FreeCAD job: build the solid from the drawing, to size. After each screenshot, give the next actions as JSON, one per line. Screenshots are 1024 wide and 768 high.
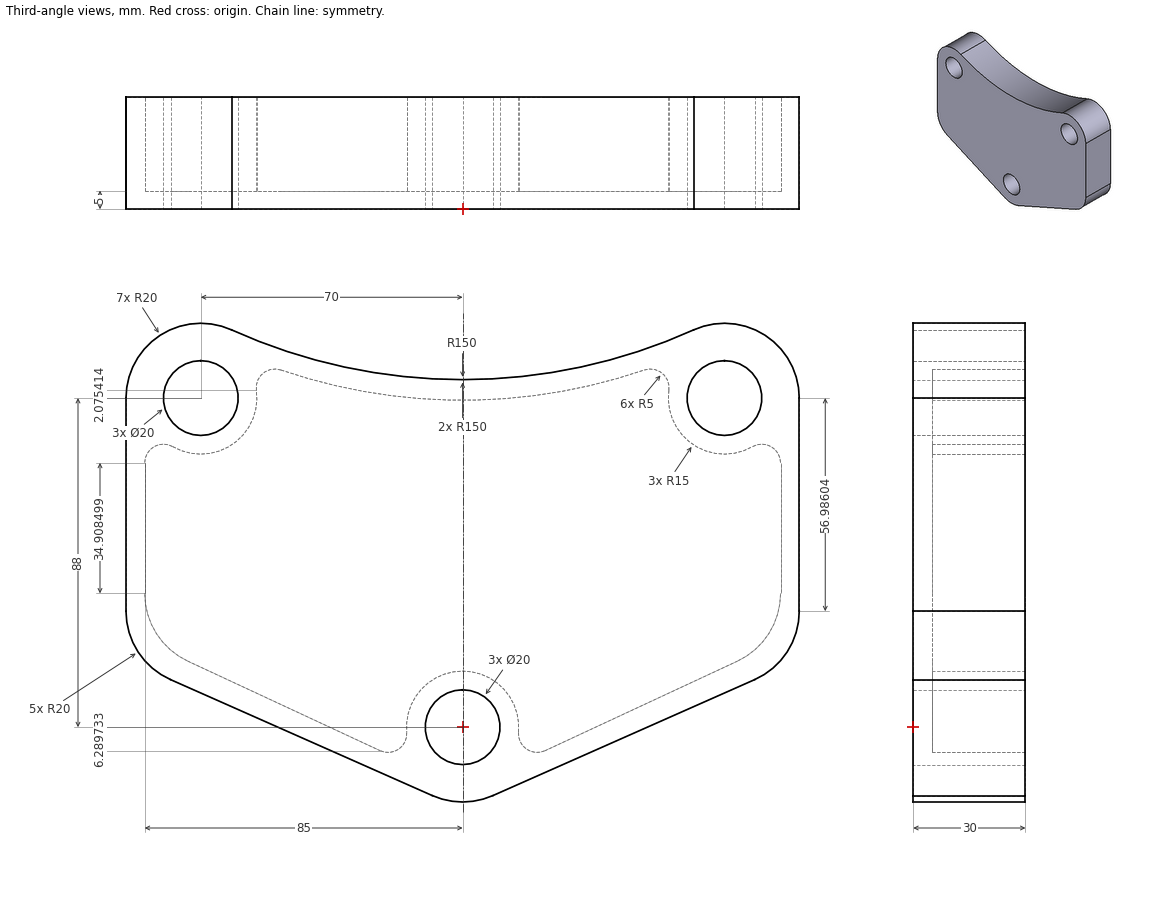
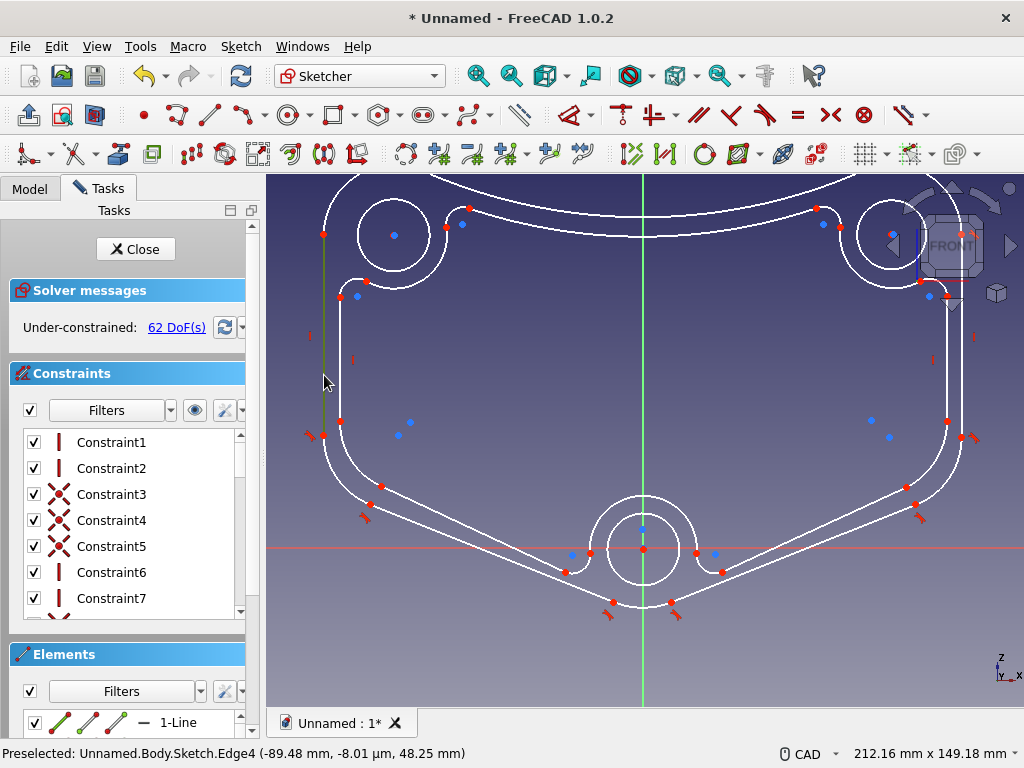
{"action": "left_click", "coordinate": [329, 208]}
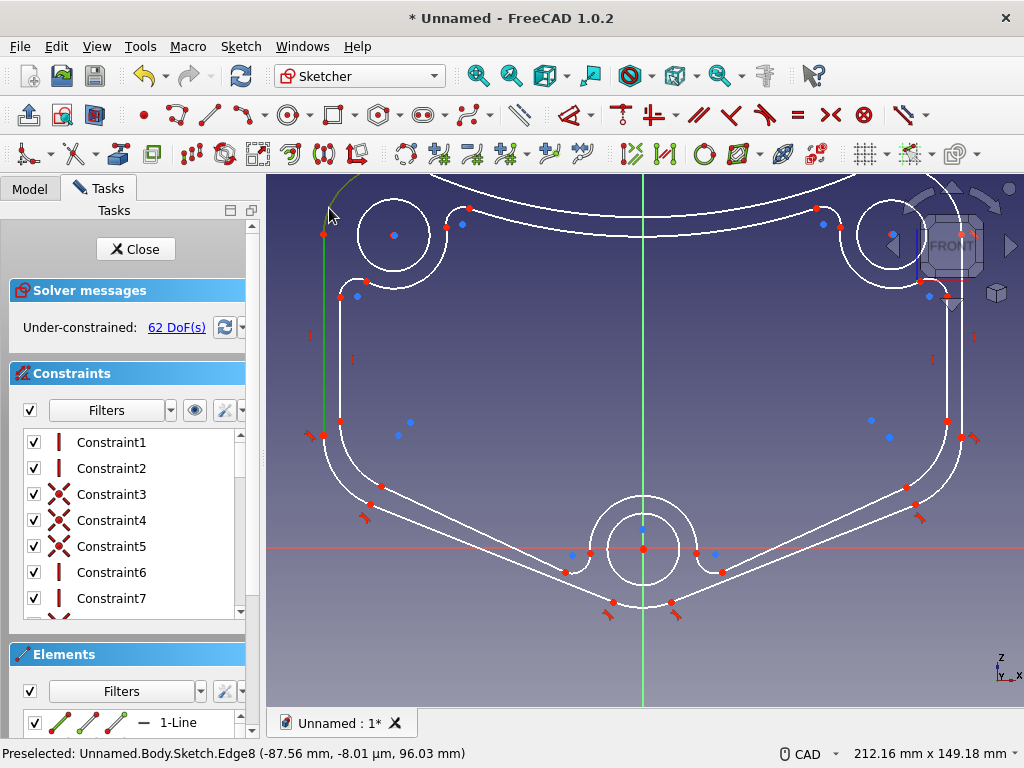
{"action": "left_click", "coordinate": [765, 116]}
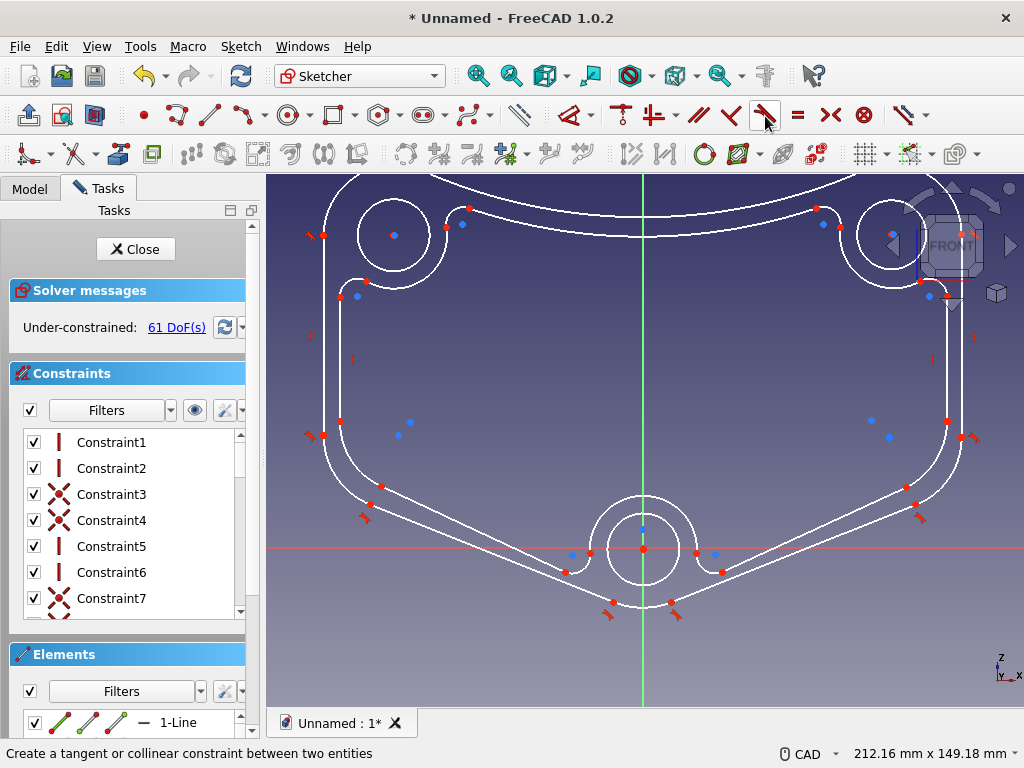
{"action": "left_click", "coordinate": [329, 209]}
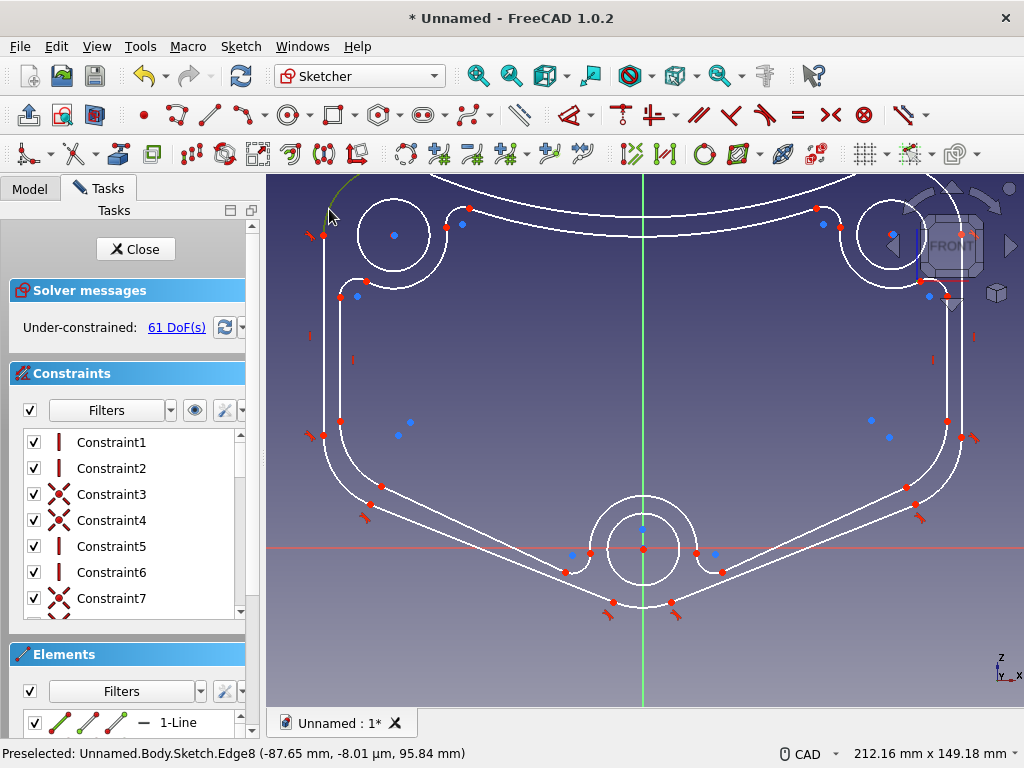
{"action": "left_click", "coordinate": [552, 210]}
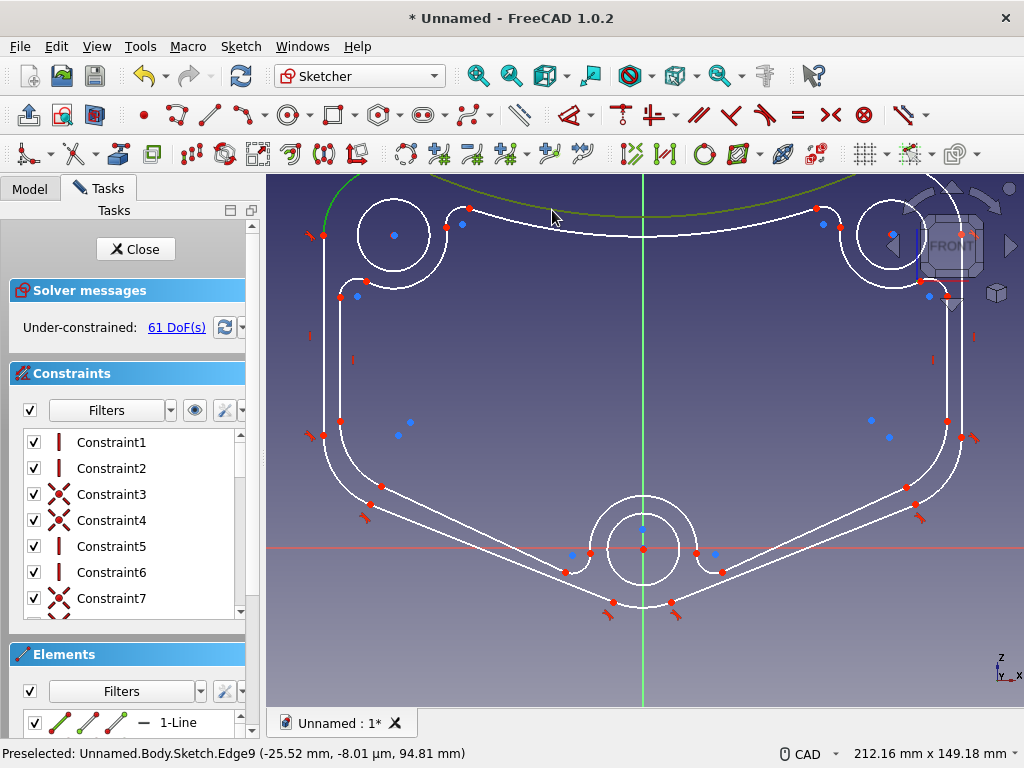
{"action": "left_click", "coordinate": [765, 116]}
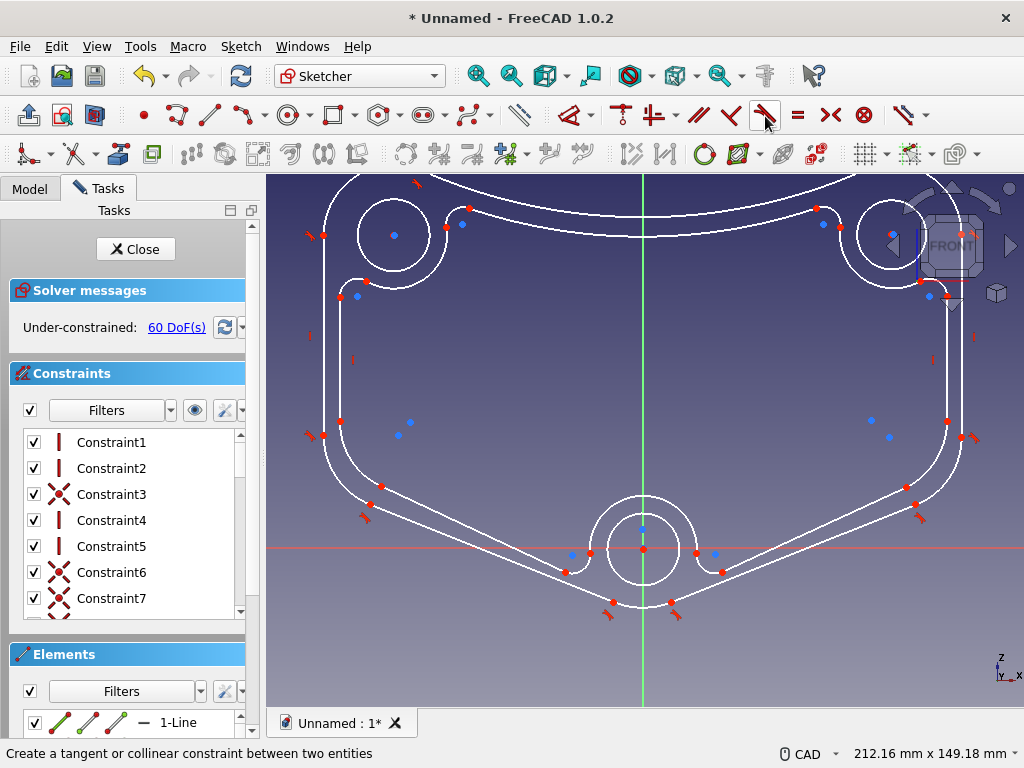
{"action": "left_click", "coordinate": [553, 210]}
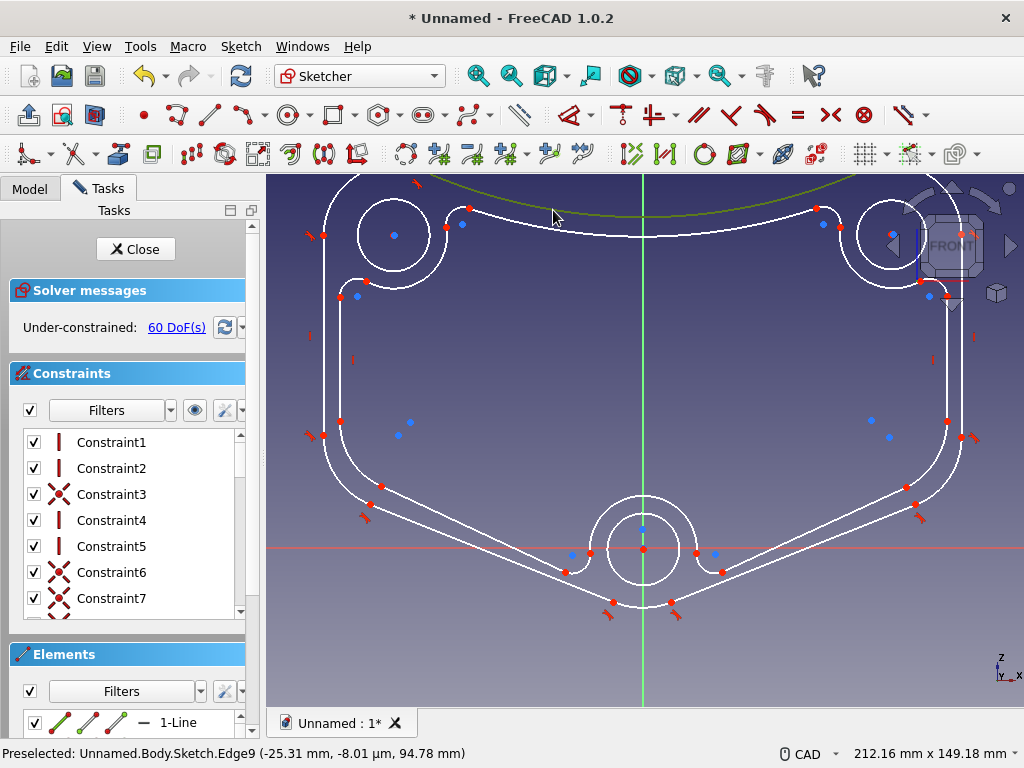
{"action": "scroll", "coordinate": [440, 534], "scroll_direction": "down", "scroll_amount": 2}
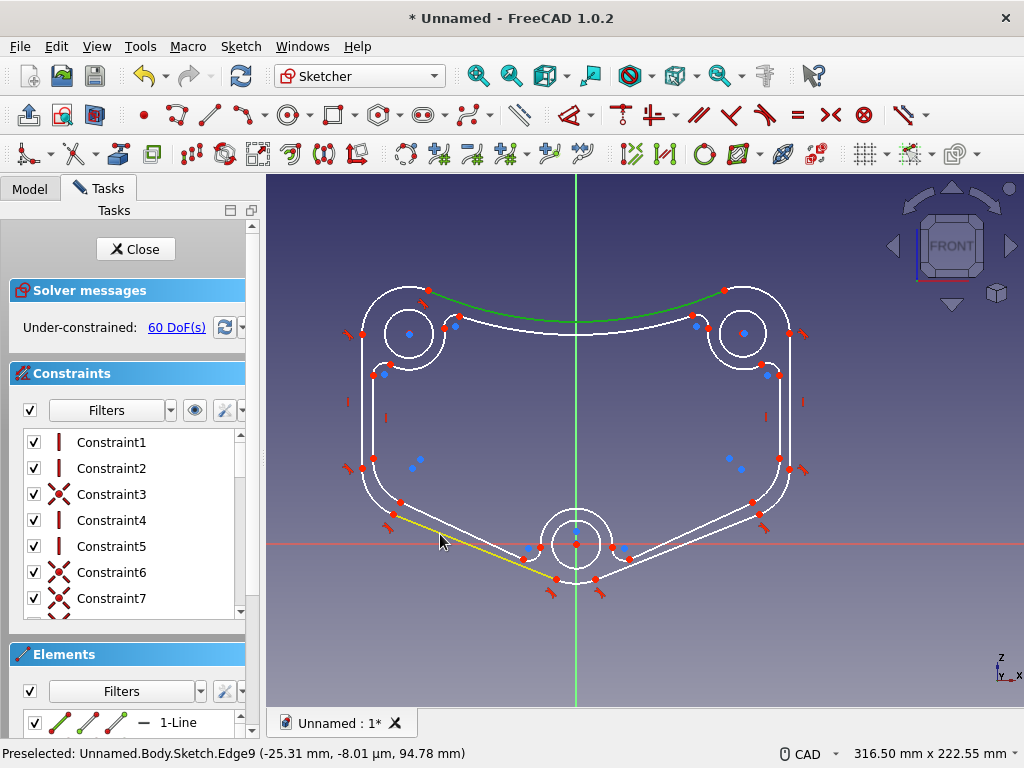
{"action": "left_click", "coordinate": [782, 307]}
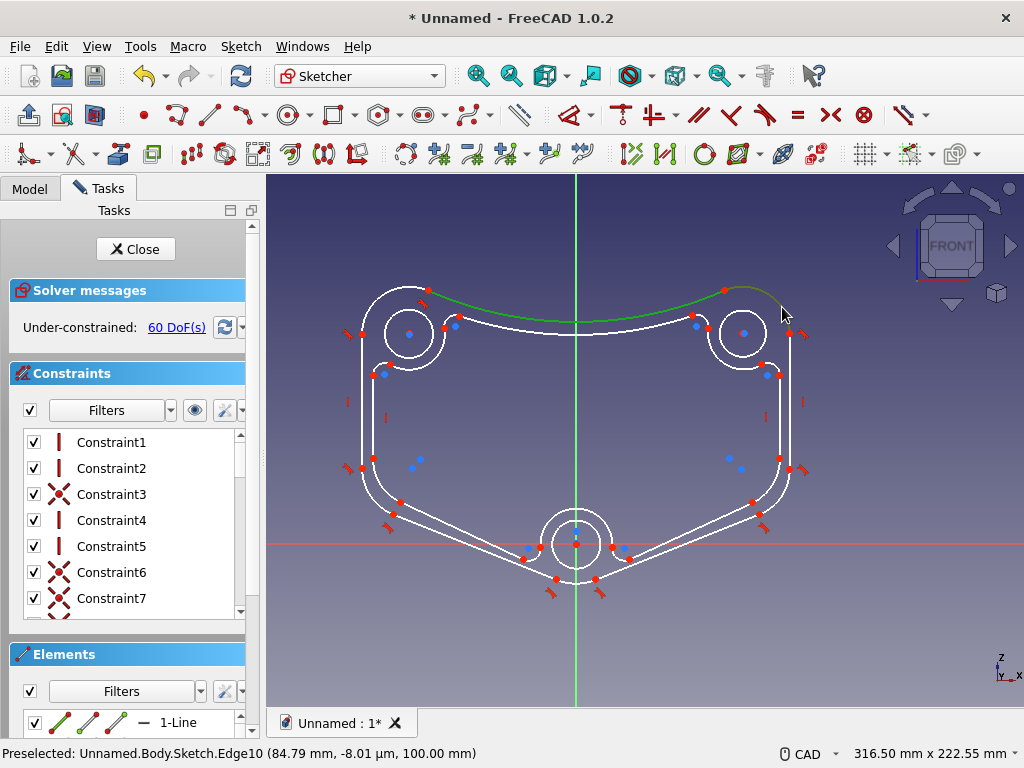
{"action": "left_click", "coordinate": [765, 116]}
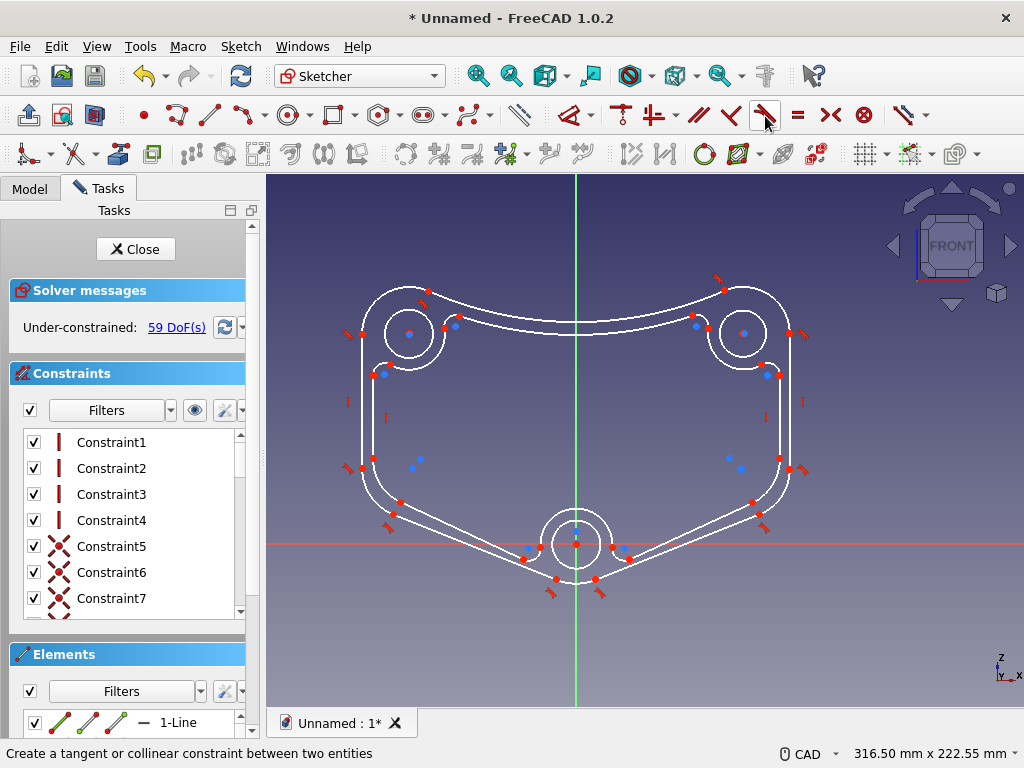
{"action": "scroll", "coordinate": [373, 400], "scroll_direction": "up", "scroll_amount": 2}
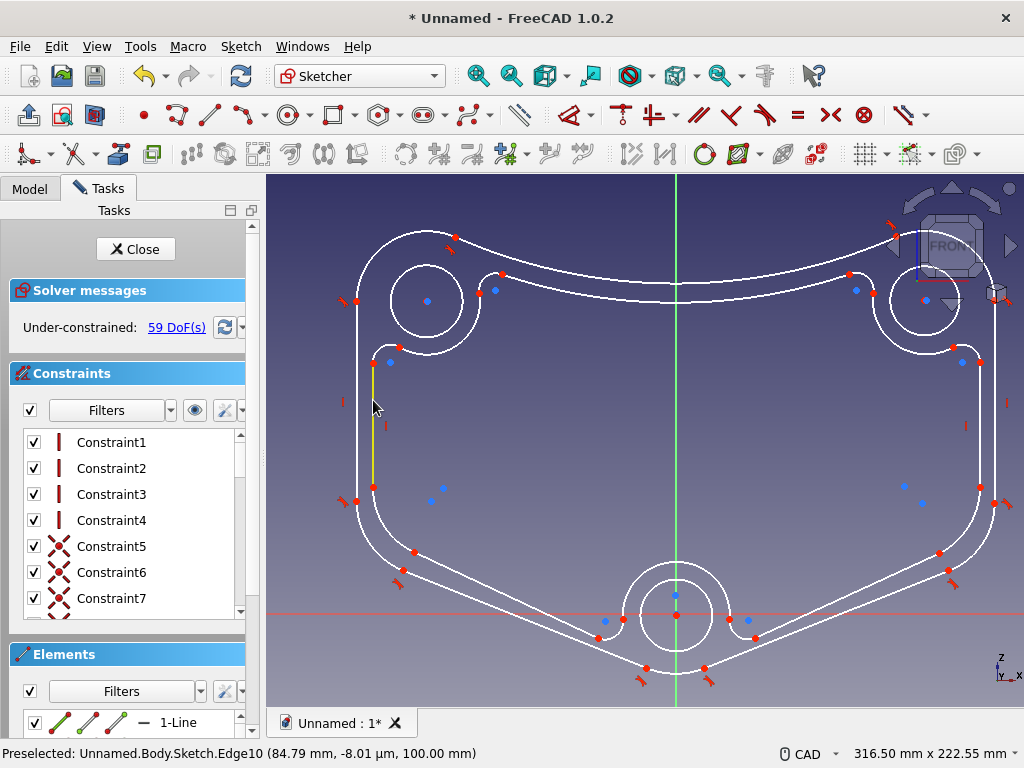
{"action": "left_click", "coordinate": [373, 400]}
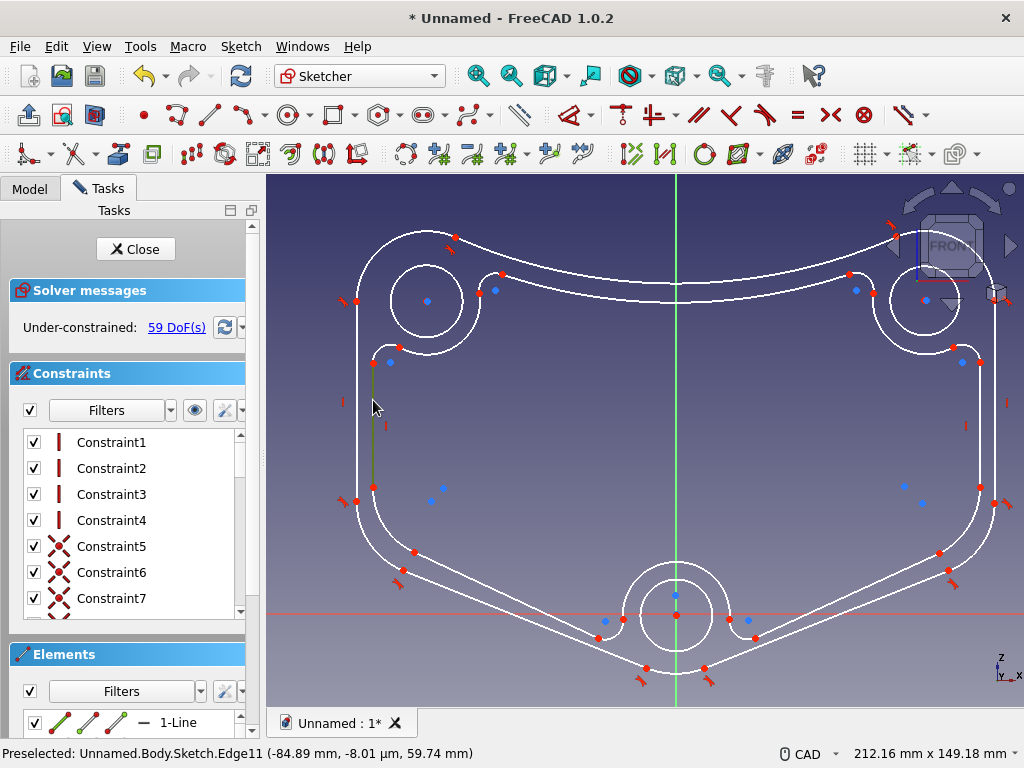
{"action": "left_click", "coordinate": [377, 511]}